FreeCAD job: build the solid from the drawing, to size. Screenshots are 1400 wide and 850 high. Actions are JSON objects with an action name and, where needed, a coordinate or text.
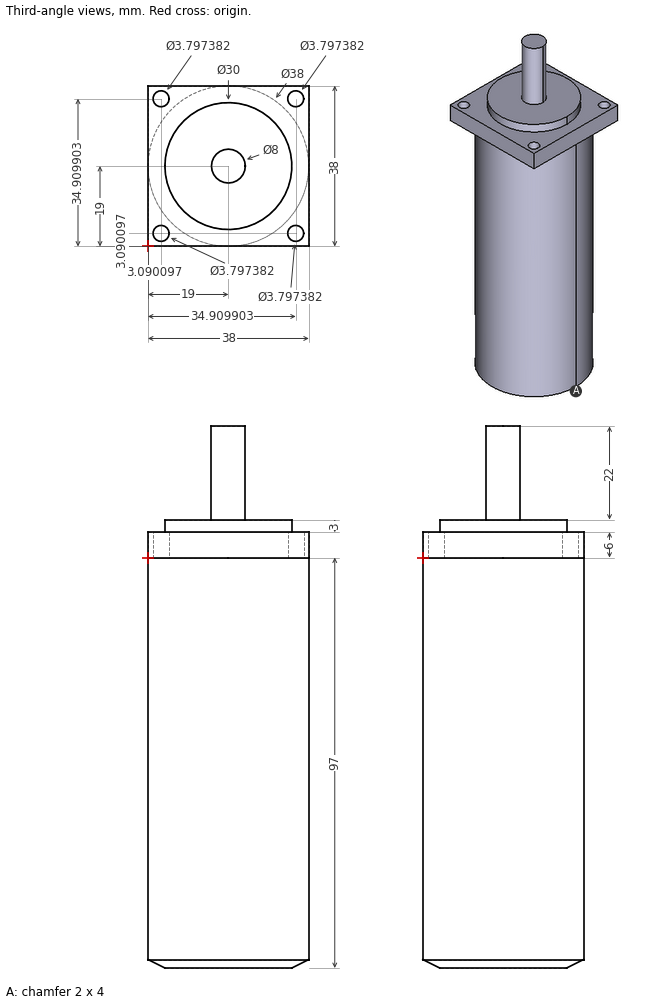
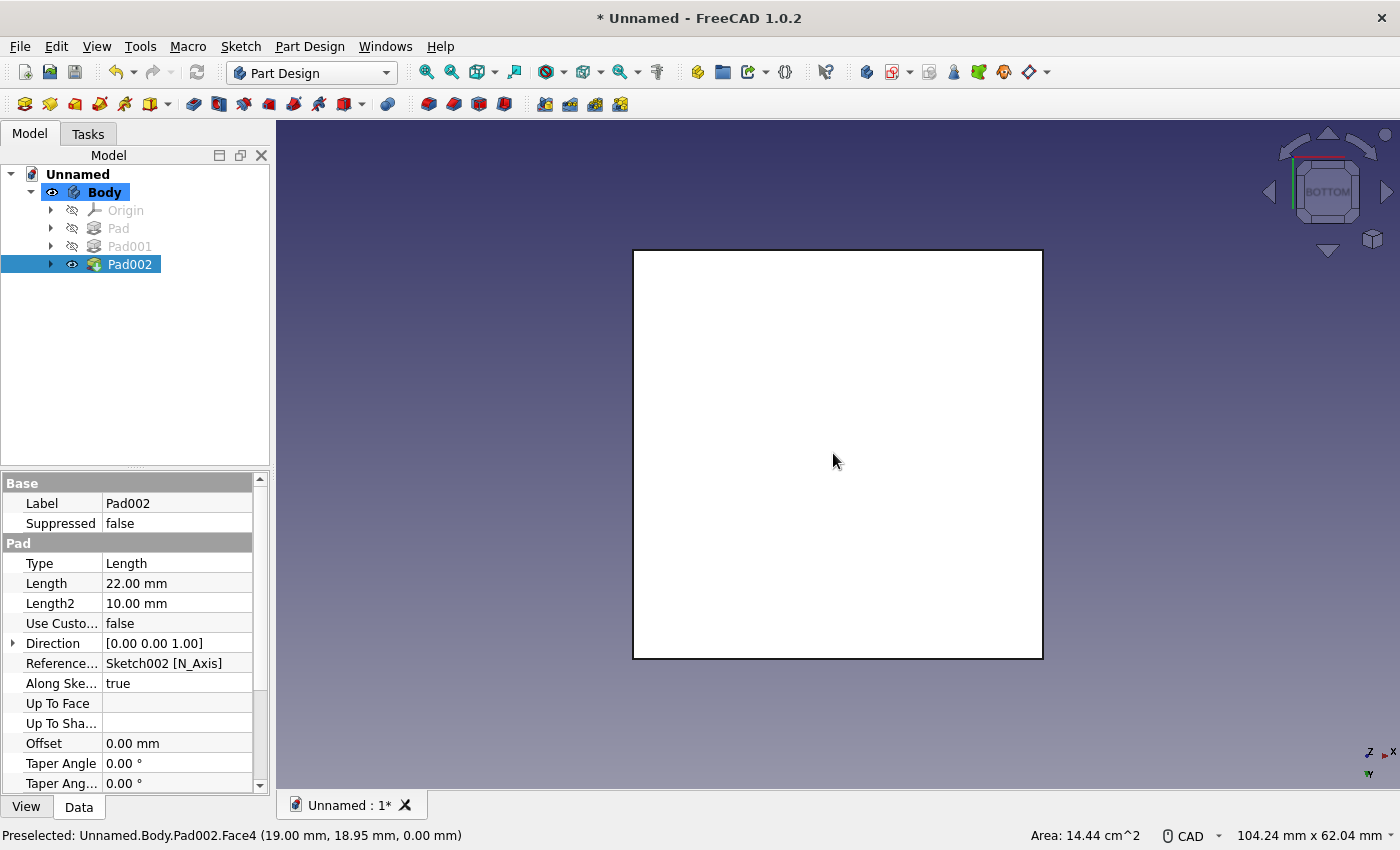
{"action": "left_click", "coordinate": [892, 72]}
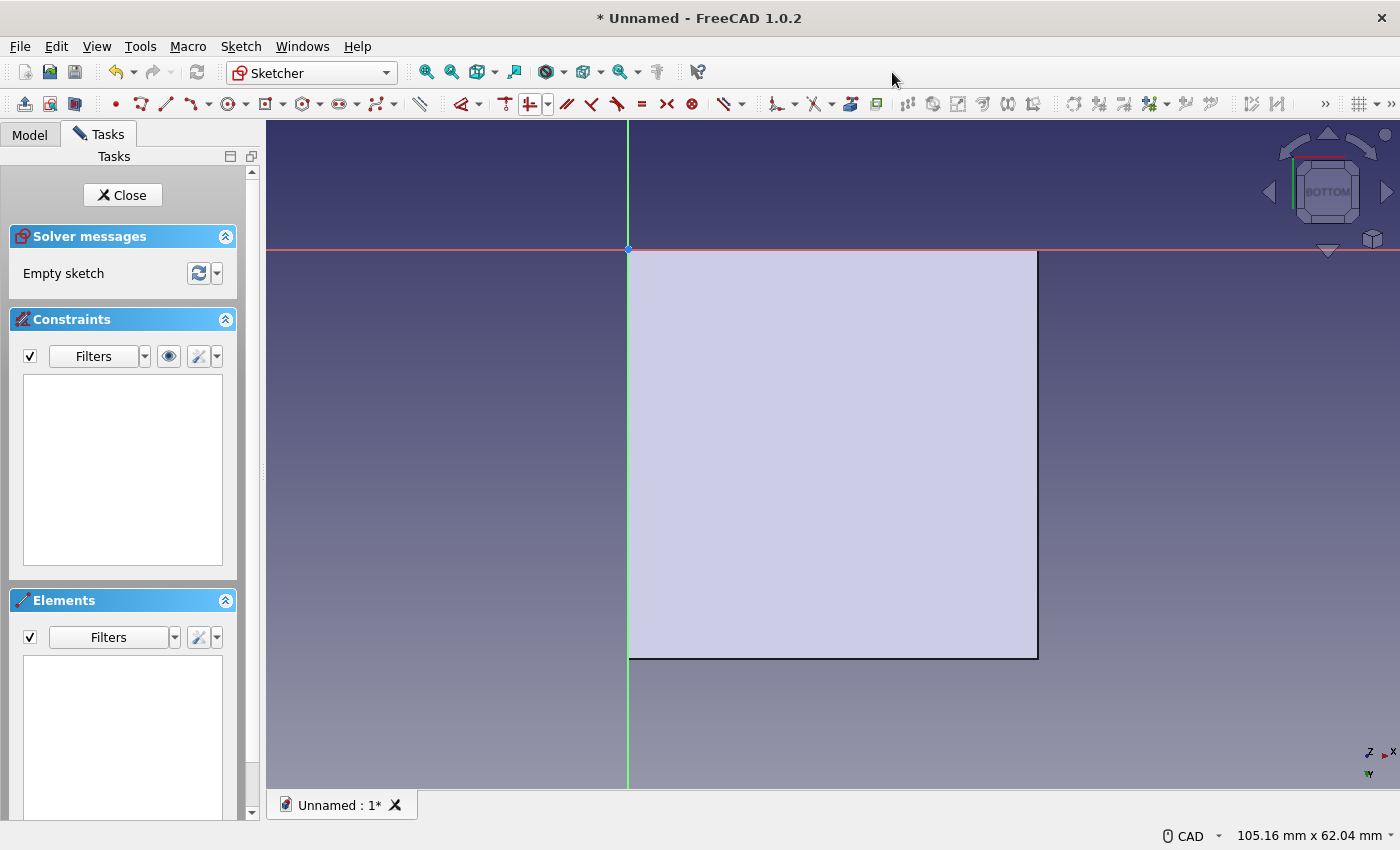
{"action": "left_click", "coordinate": [228, 104]}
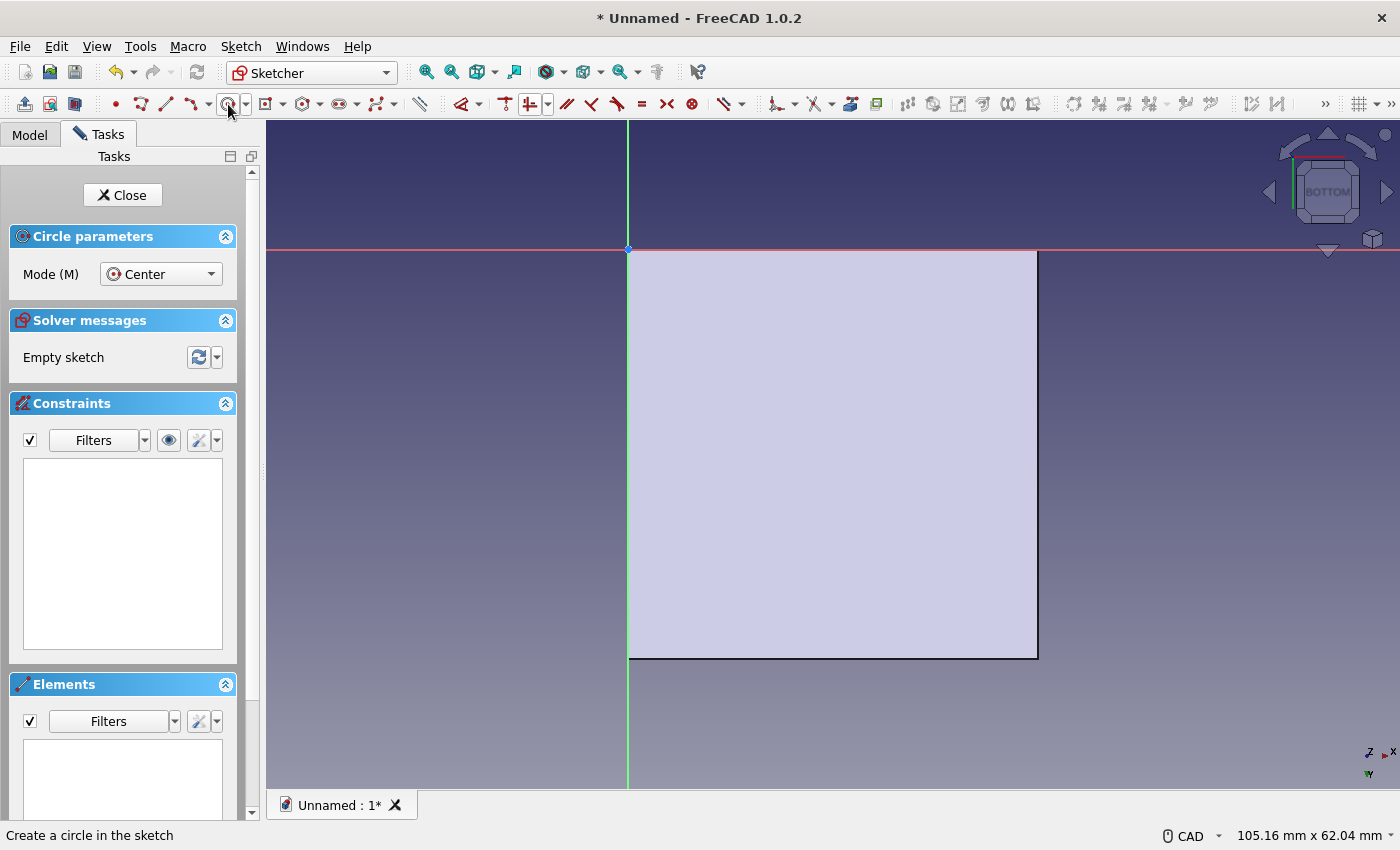
{"action": "left_click", "coordinate": [833, 454]}
{"action": "mouse_move", "coordinate": [978, 310]}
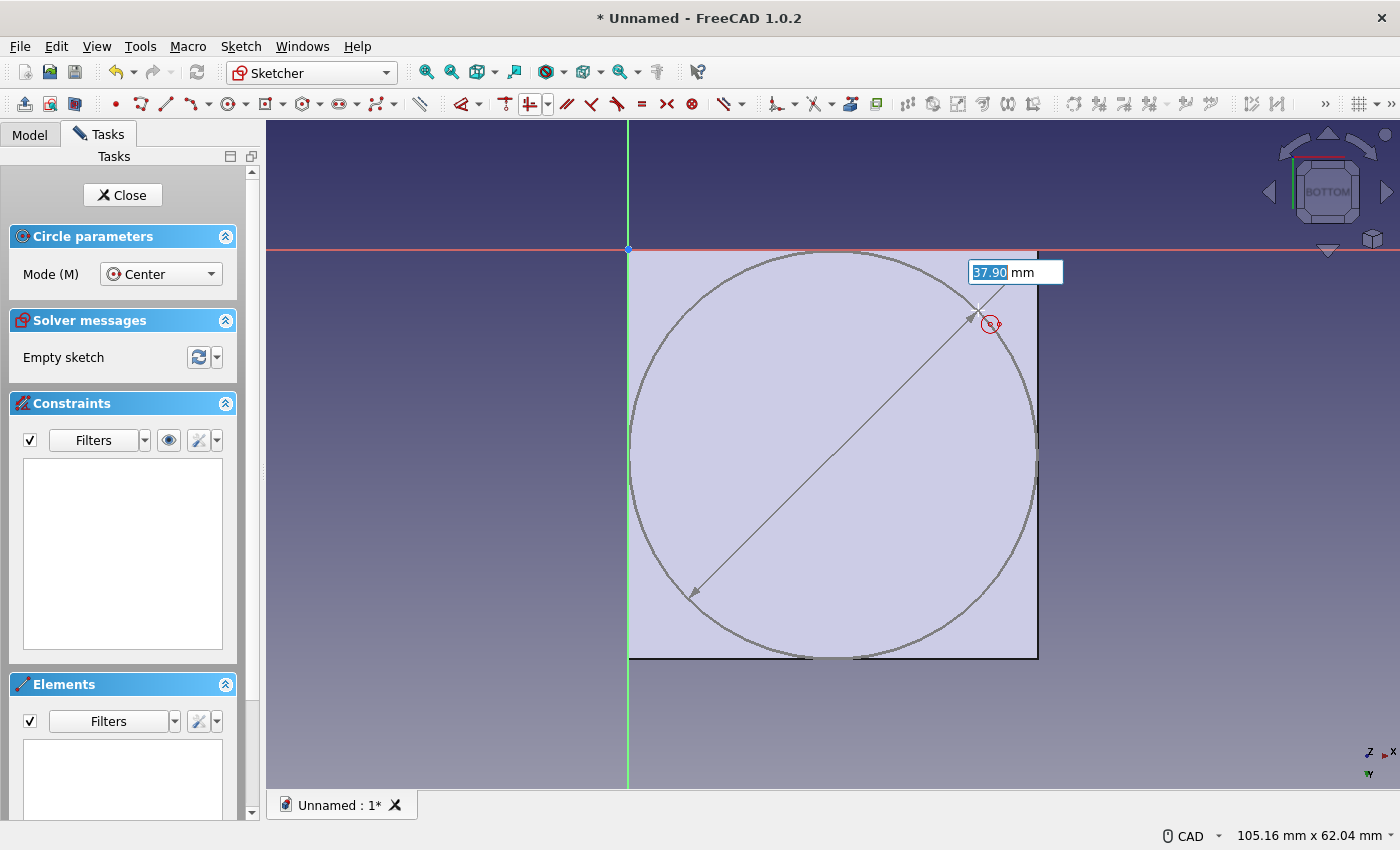
{"action": "type", "text": "38"}
{"action": "key", "text": "Return"}
{"action": "key", "text": "Escape"}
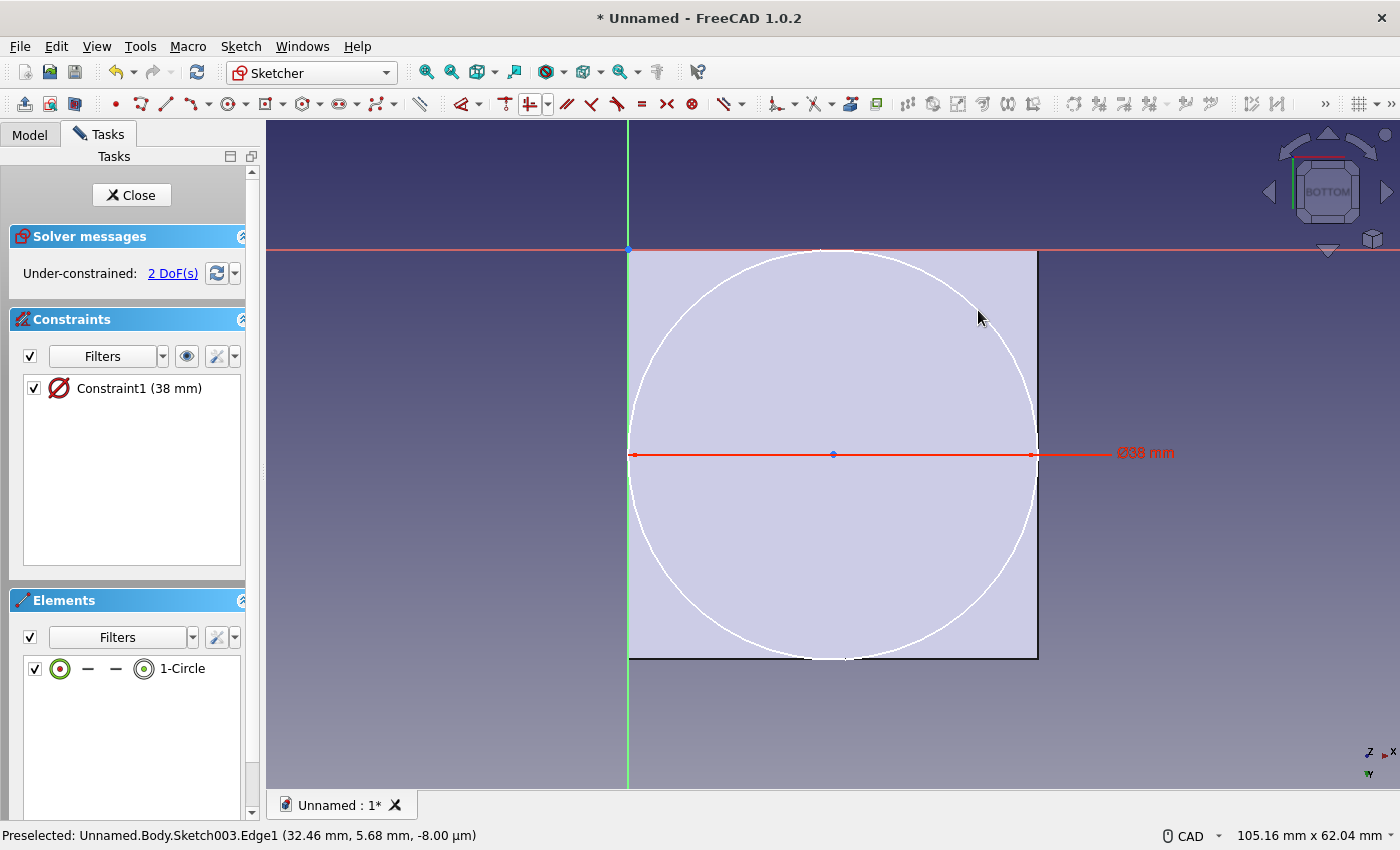
{"action": "left_click", "coordinate": [460, 104]}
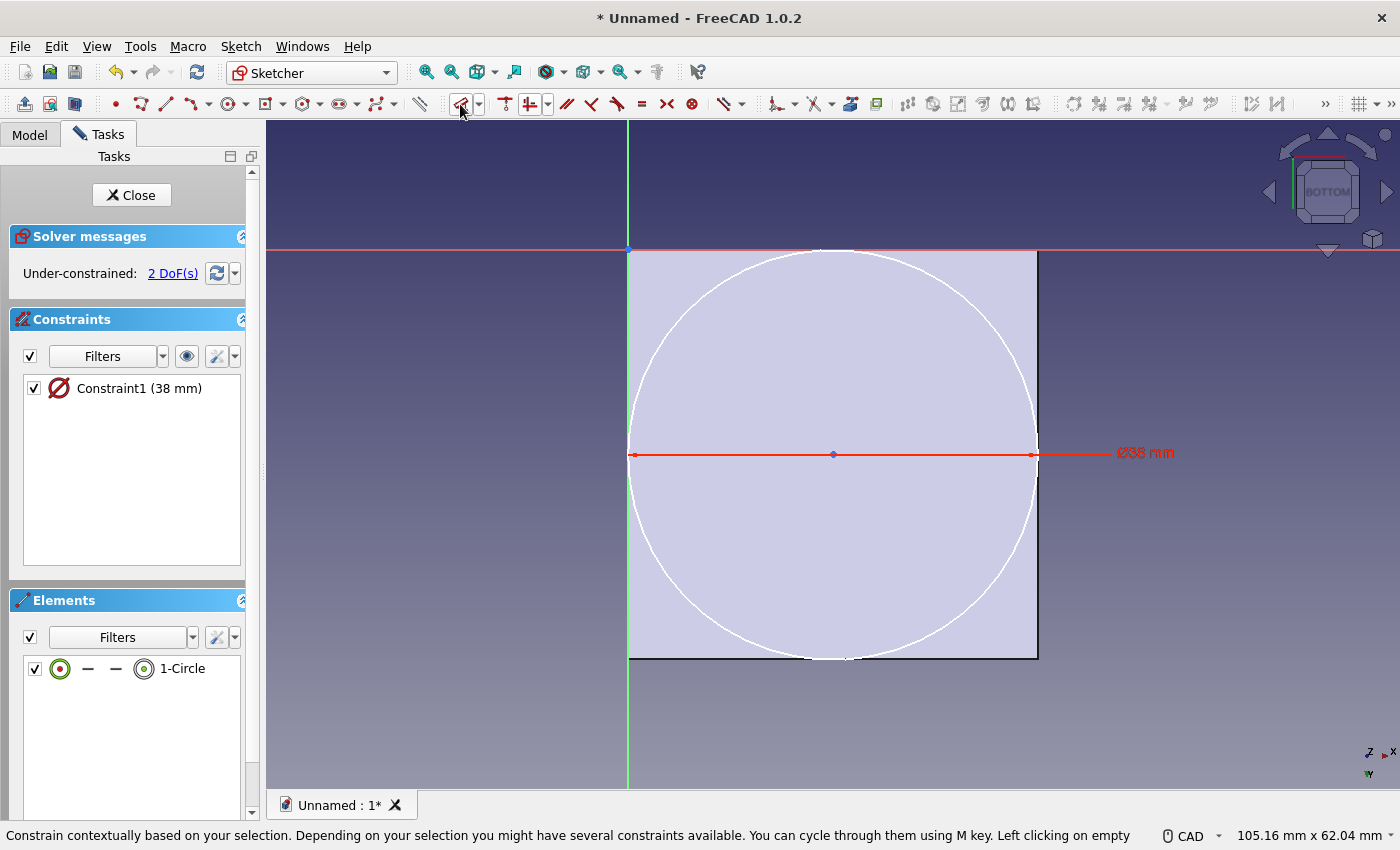
{"action": "left_click", "coordinate": [833, 455]}
{"action": "left_click", "coordinate": [731, 216]}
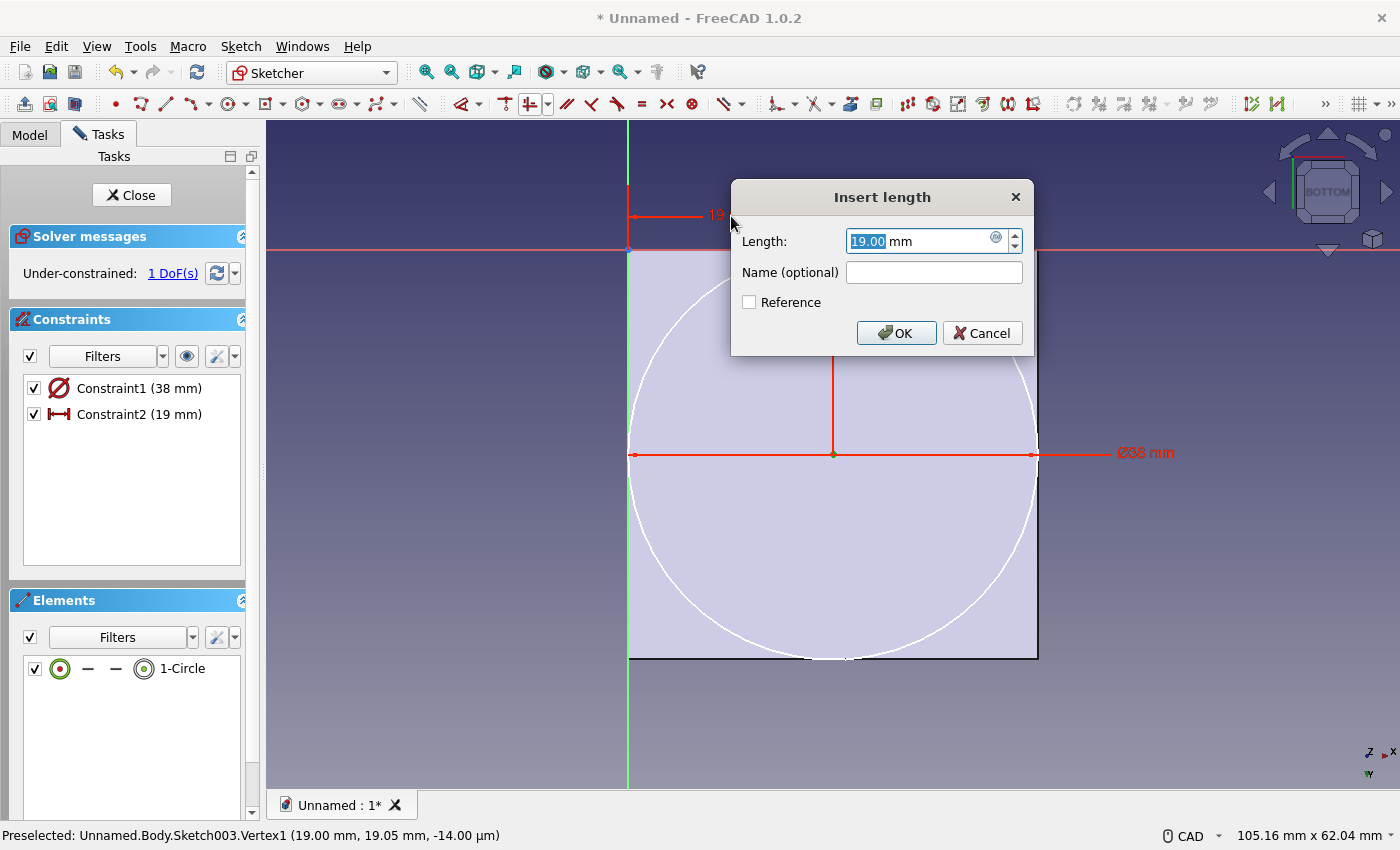
{"action": "type", "text": "19"}
{"action": "key", "text": "Return"}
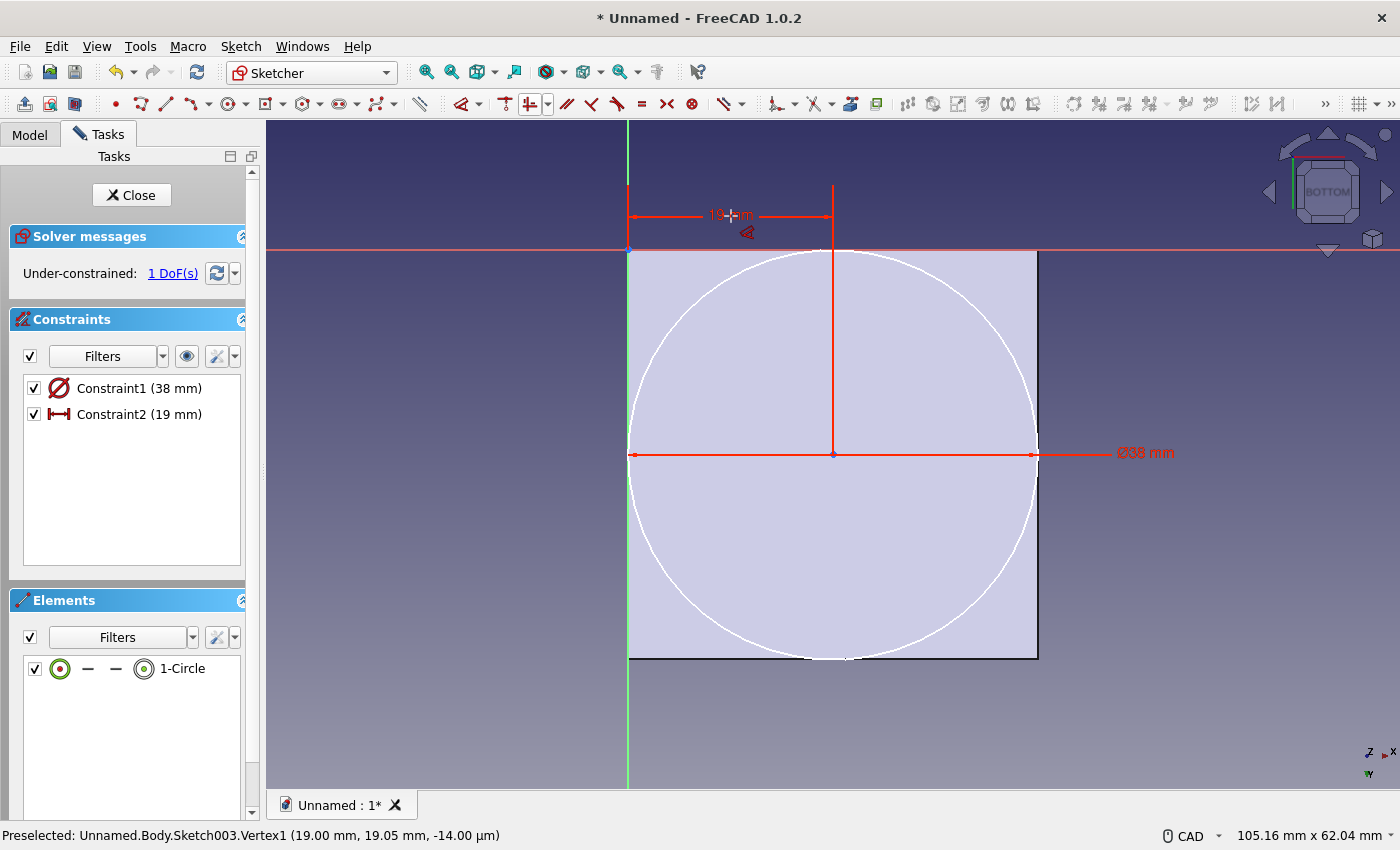
{"action": "left_click", "coordinate": [833, 455]}
{"action": "left_click", "coordinate": [594, 352]}